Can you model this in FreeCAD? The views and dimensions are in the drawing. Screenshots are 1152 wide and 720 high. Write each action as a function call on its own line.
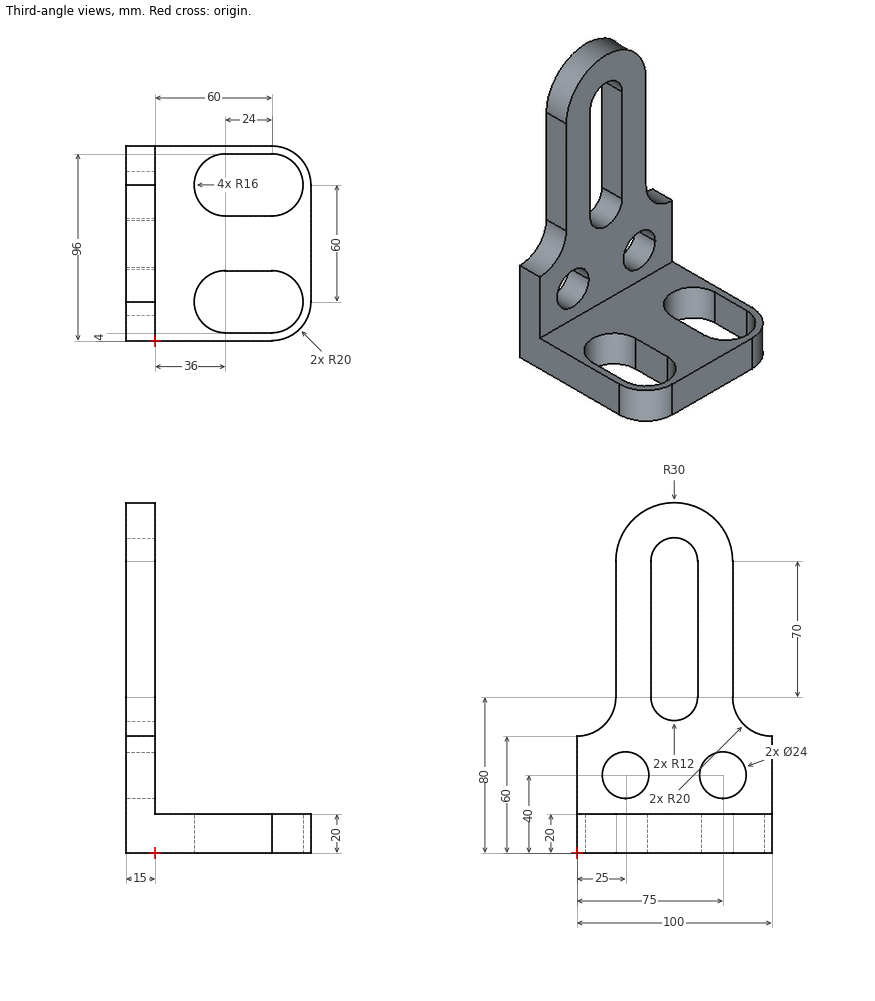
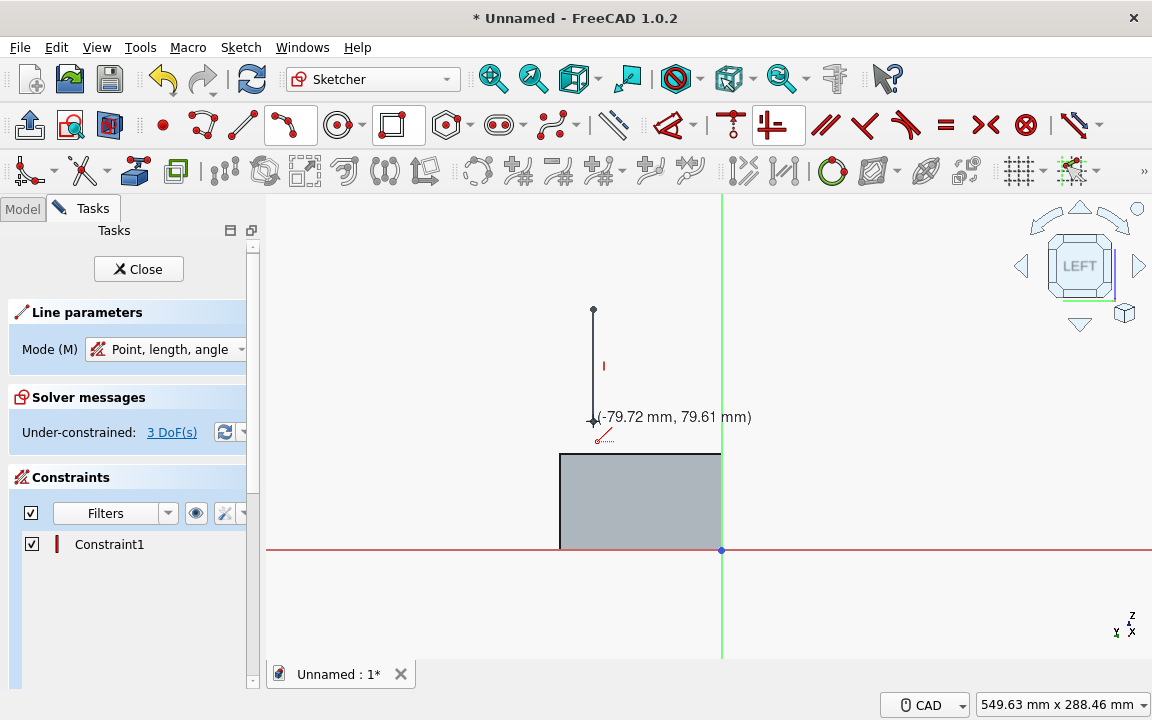
click(560, 454)
click(722, 454)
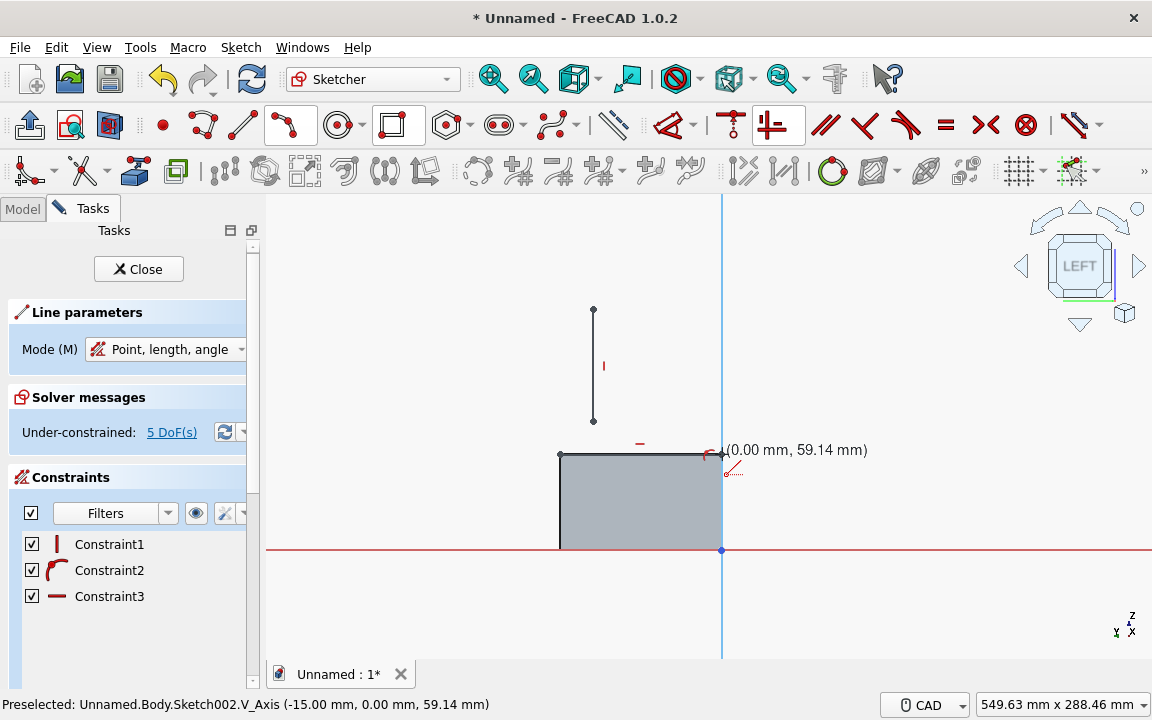
click(689, 421)
click(689, 309)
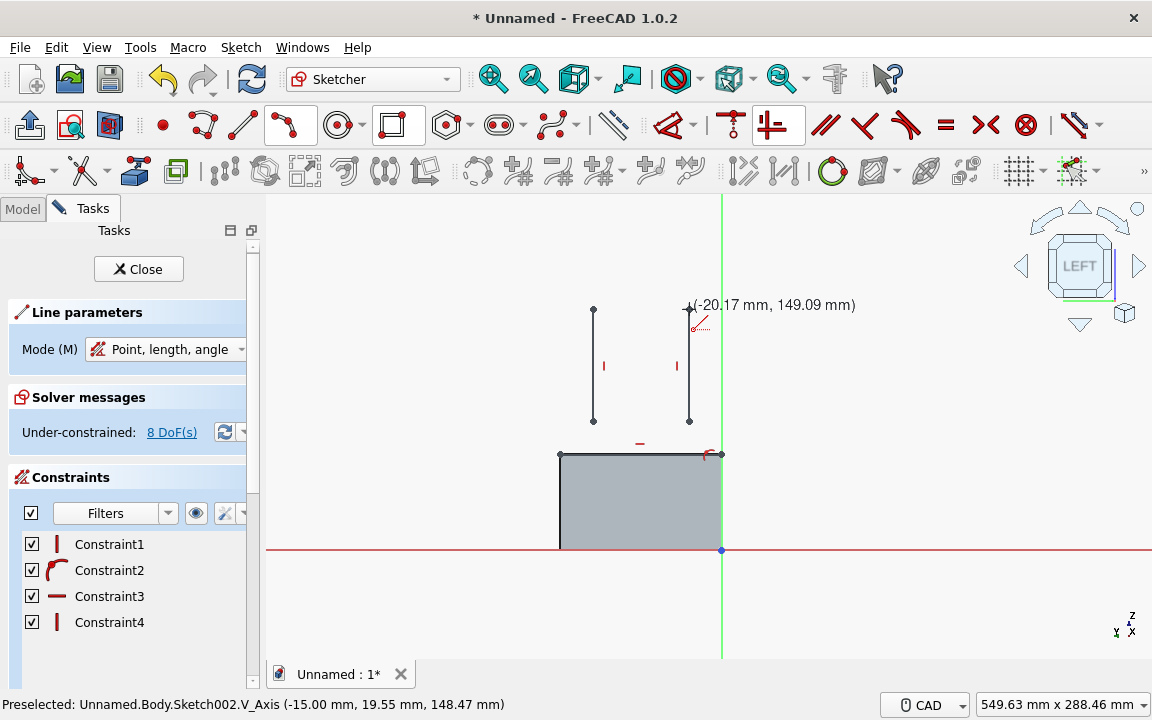
click(284, 126)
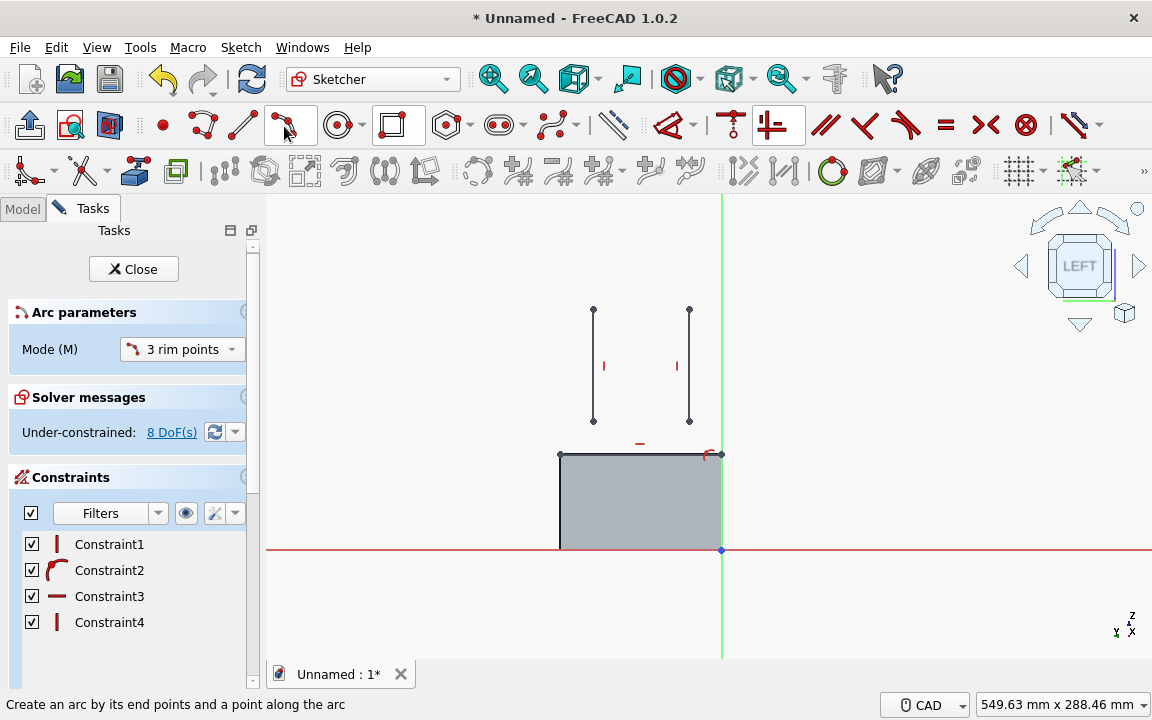
click(593, 422)
click(560, 455)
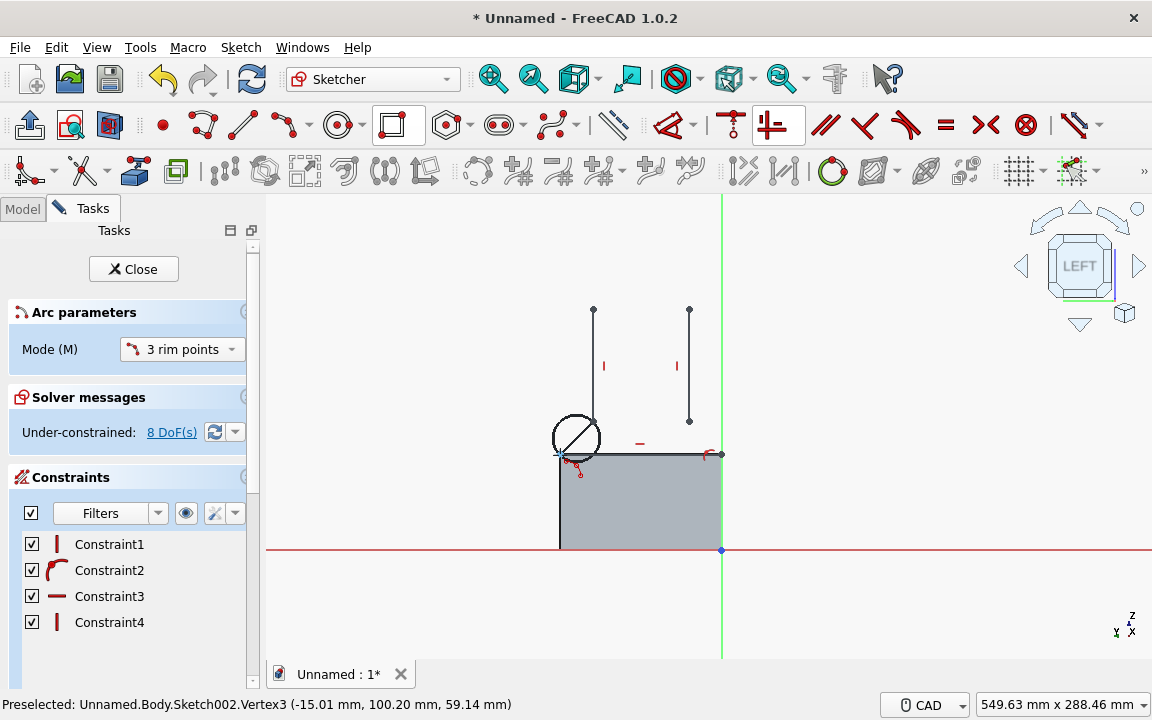
scroll(583, 444, up, 3)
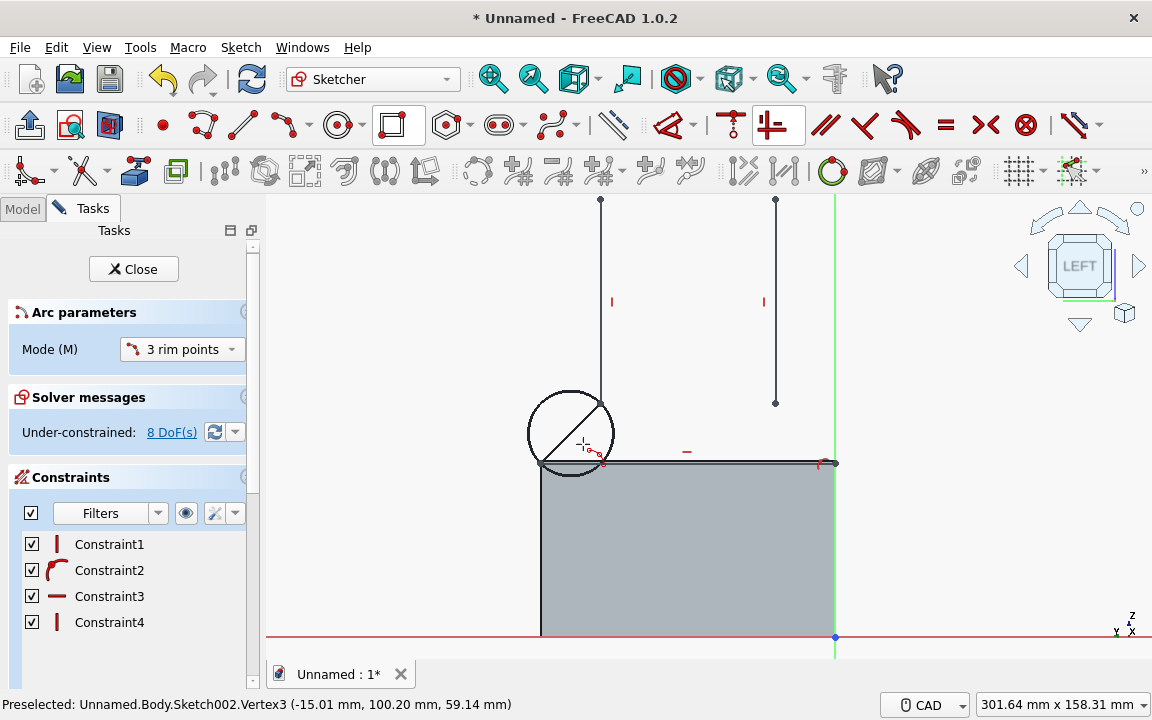
click(583, 444)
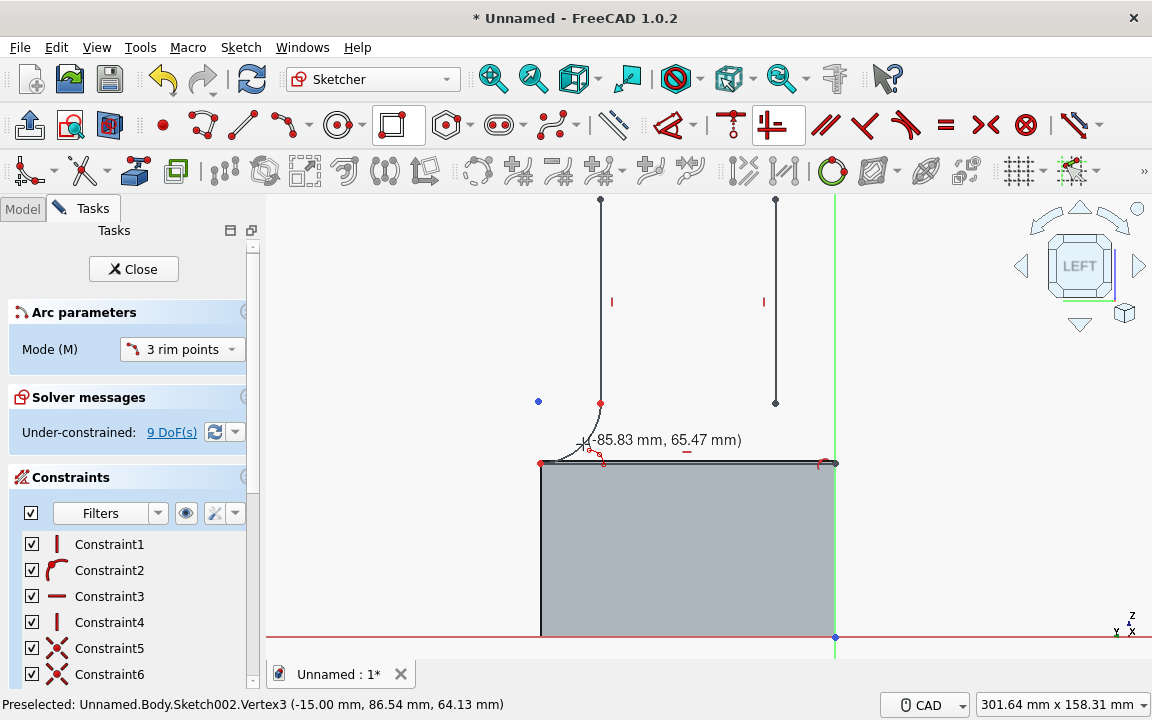
click(835, 464)
click(776, 403)
click(794, 444)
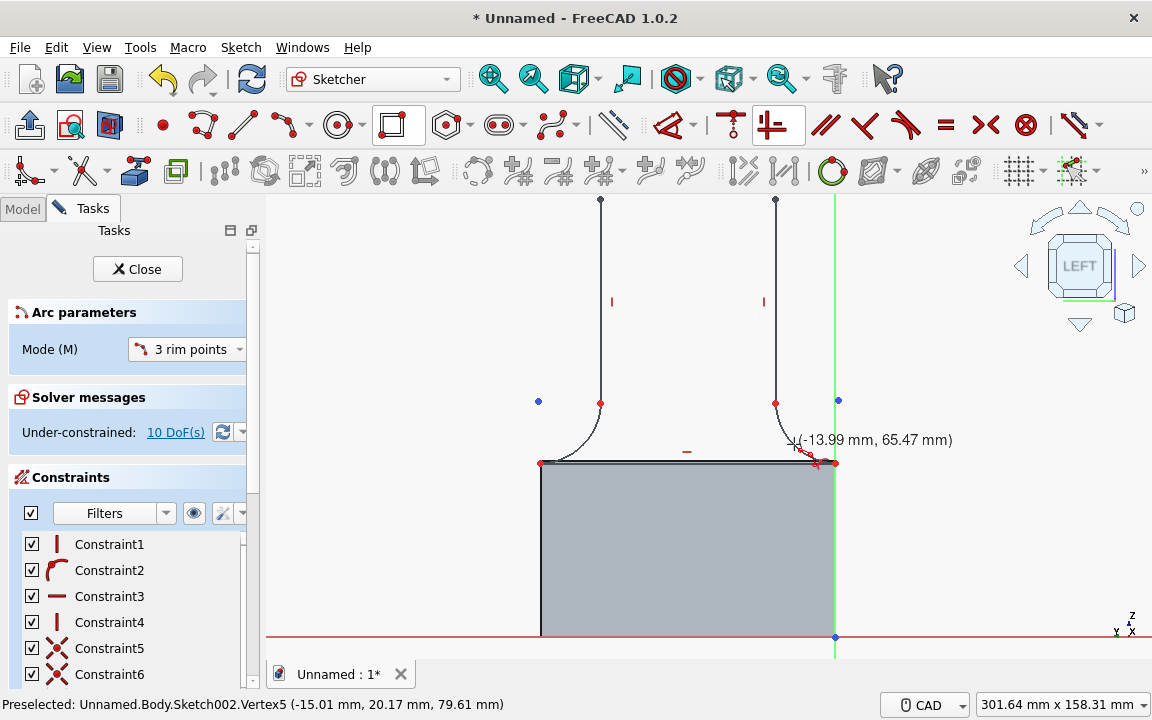
scroll(582, 492, down, 3)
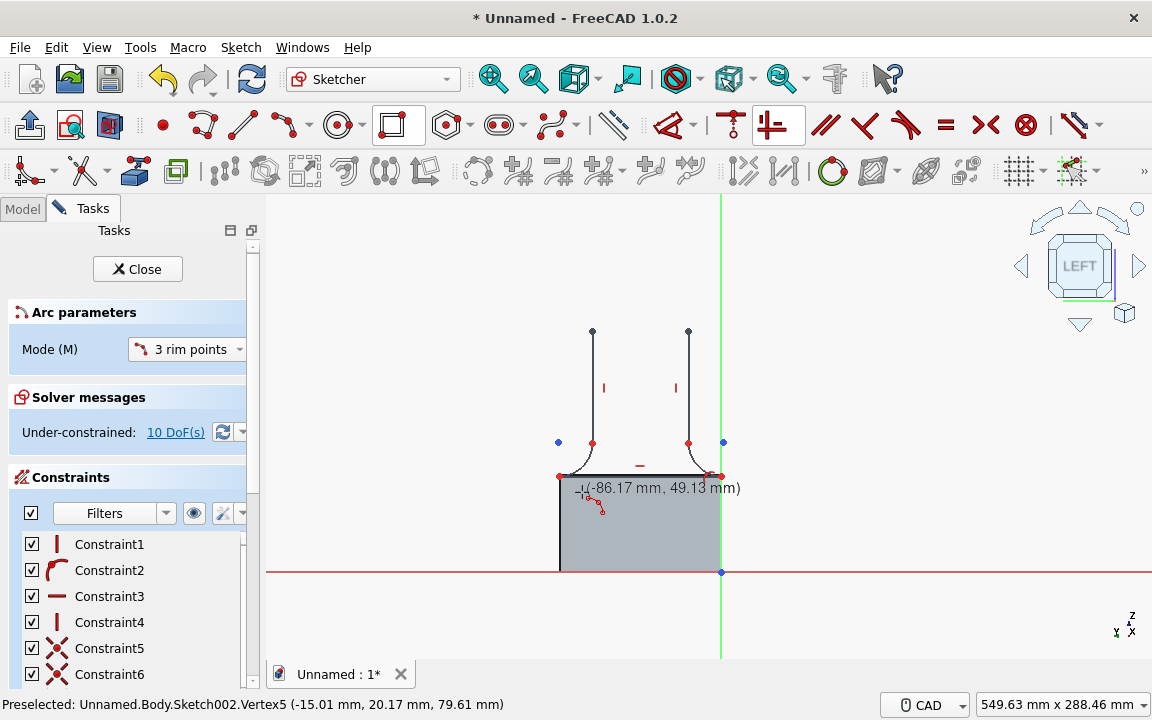
click(689, 332)
click(593, 332)
click(640, 282)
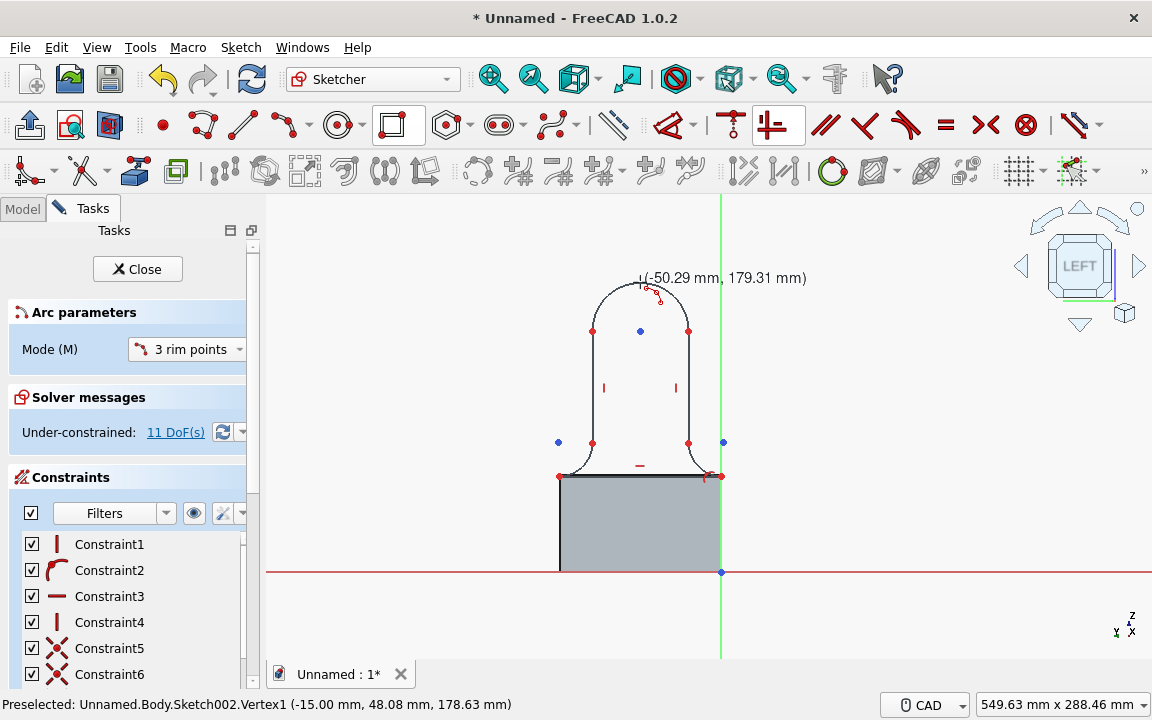
click(500, 126)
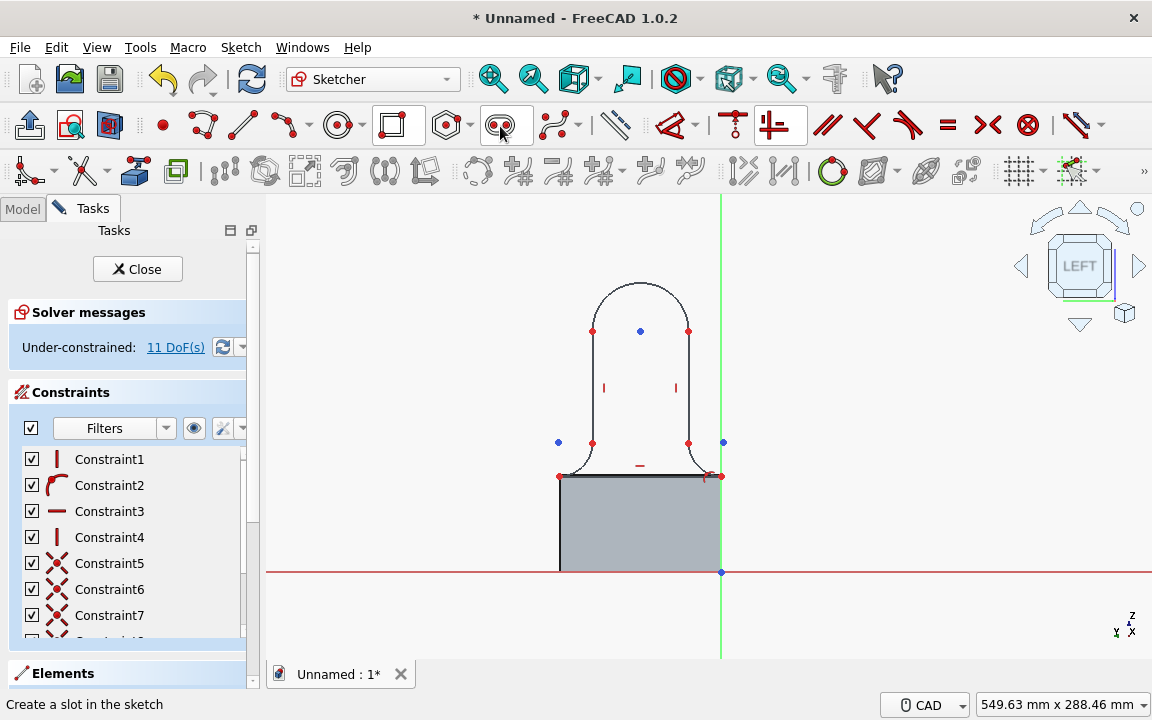
click(640, 443)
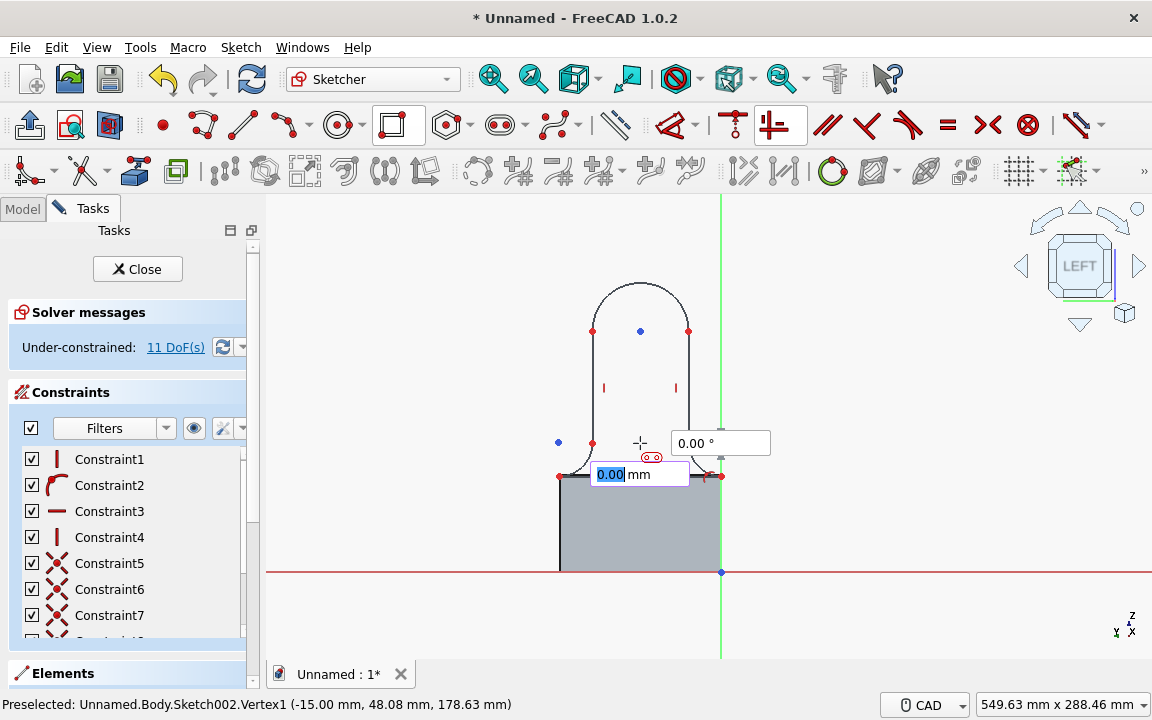
click(640, 330)